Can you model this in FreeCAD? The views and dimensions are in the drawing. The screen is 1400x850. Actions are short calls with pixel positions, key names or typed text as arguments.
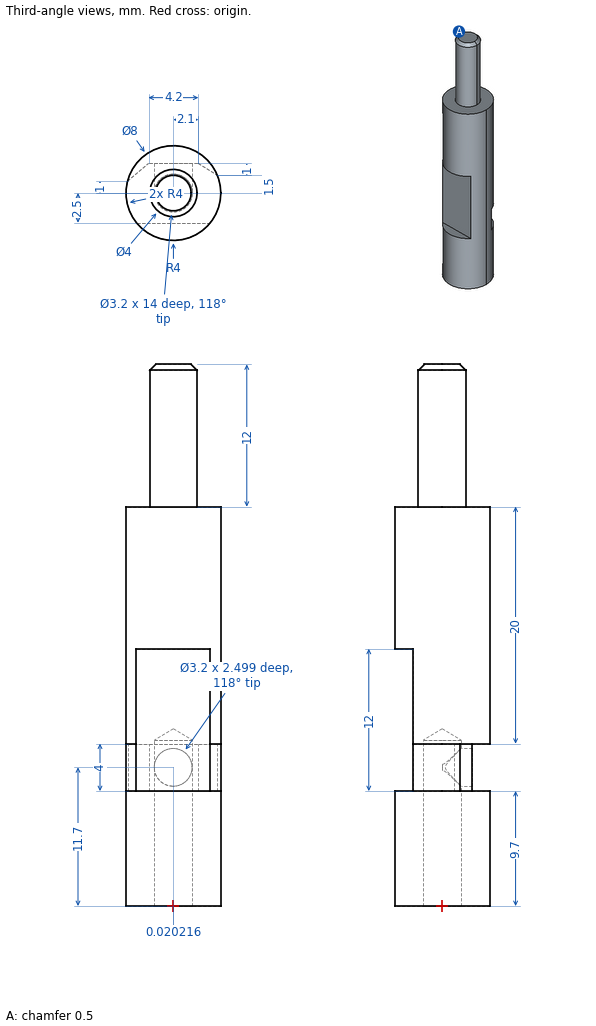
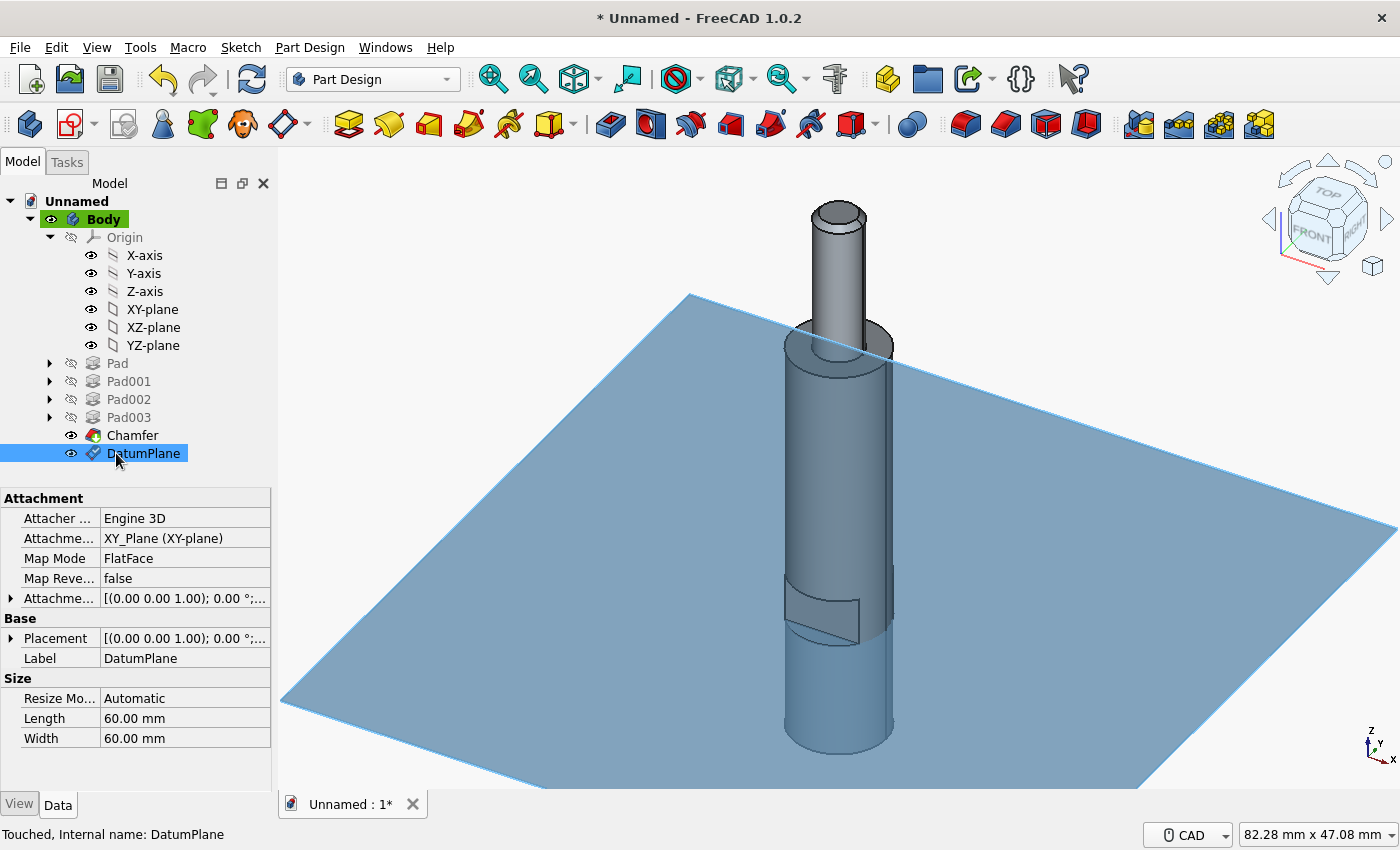
click(70, 124)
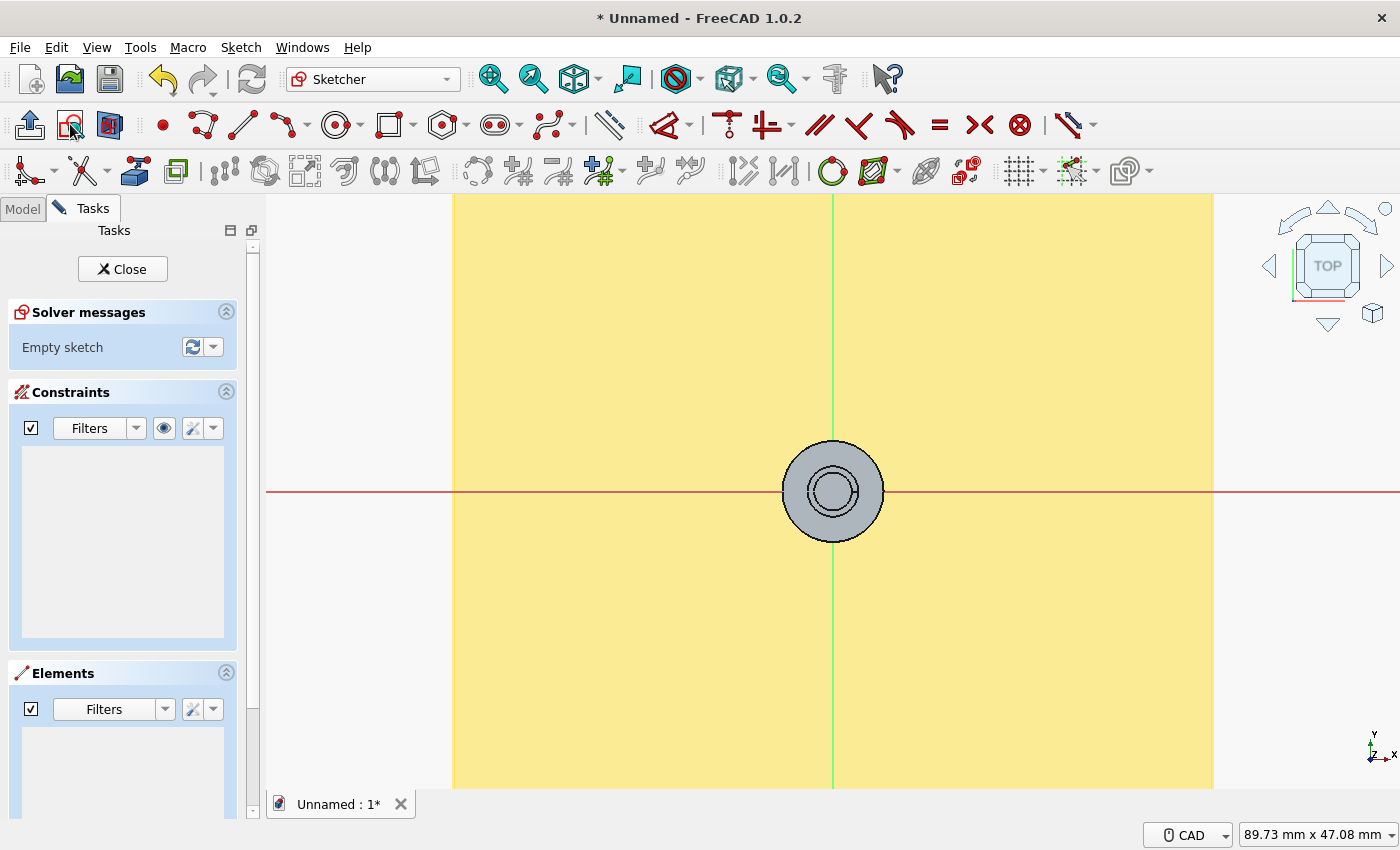
click(110, 126)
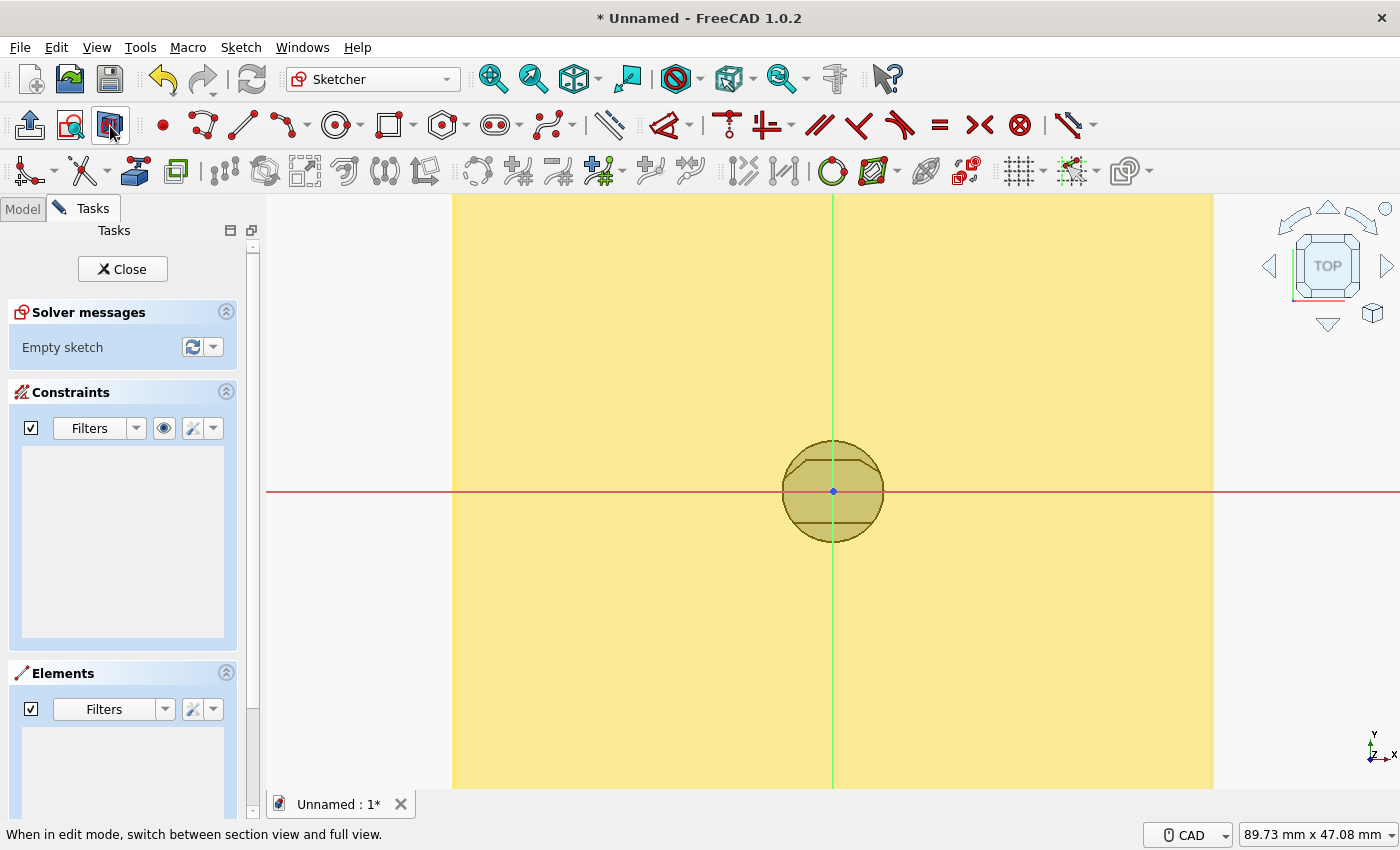
scroll(844, 521, up, 10)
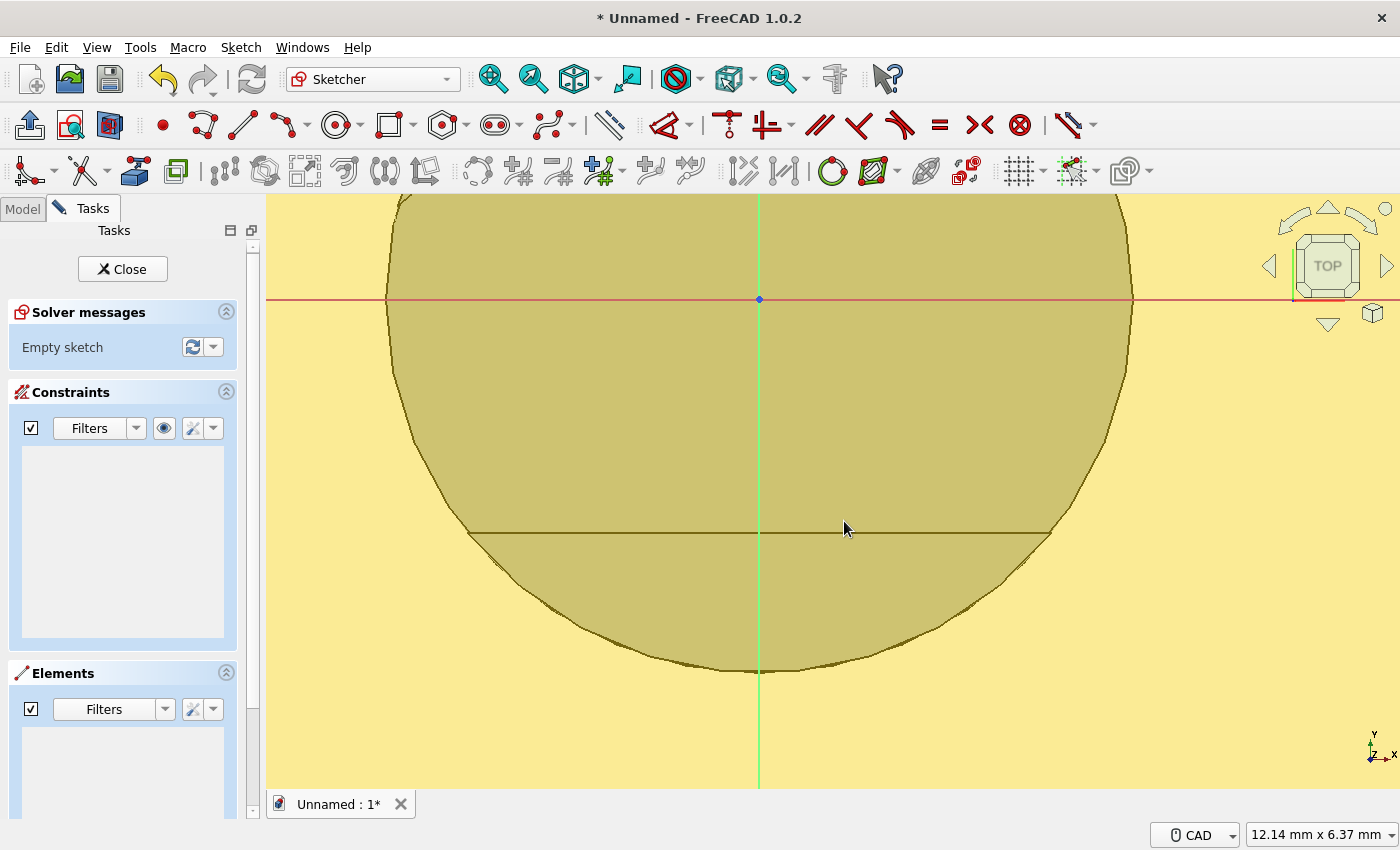
key(g)
key(l)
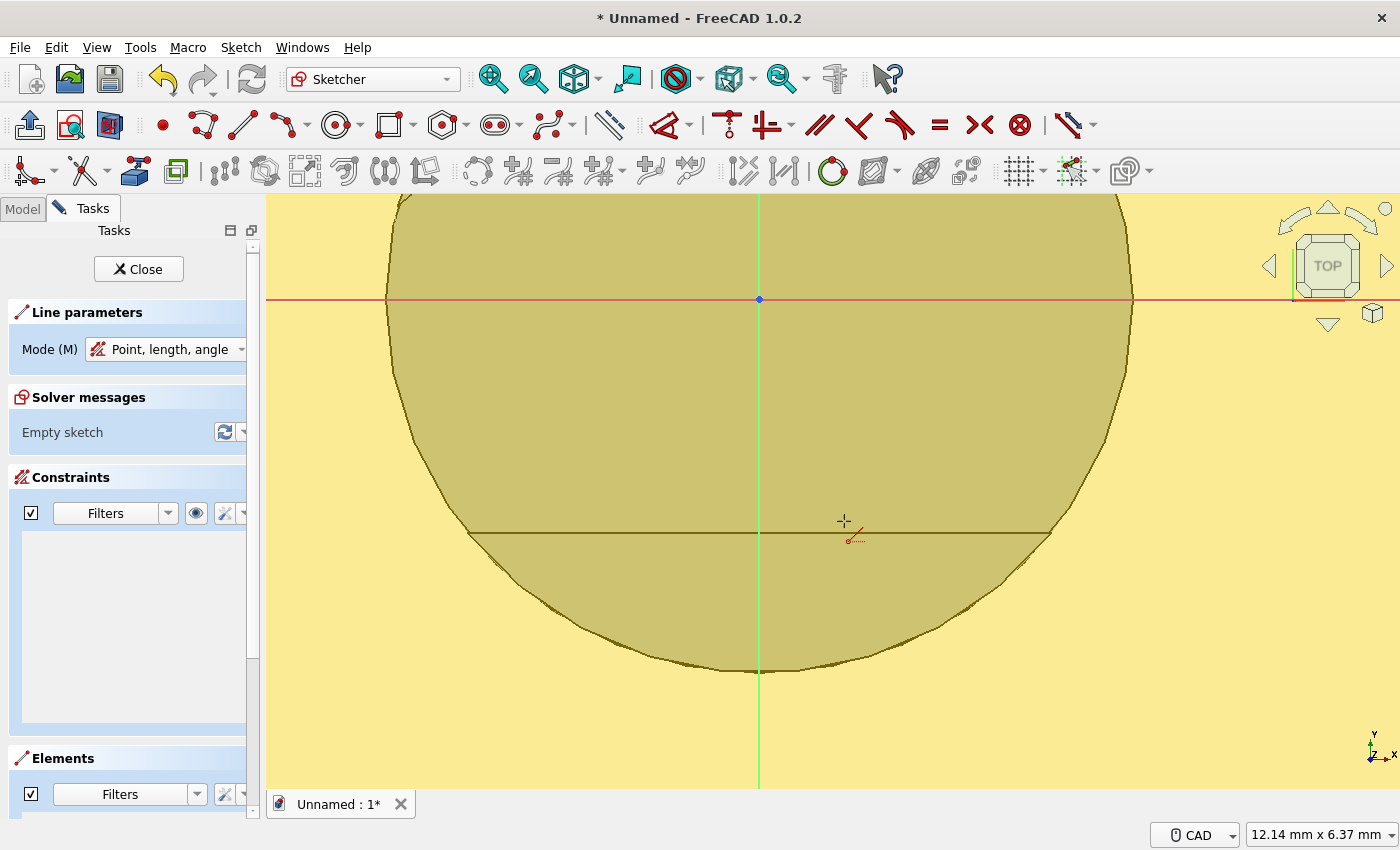
click(1051, 533)
click(468, 533)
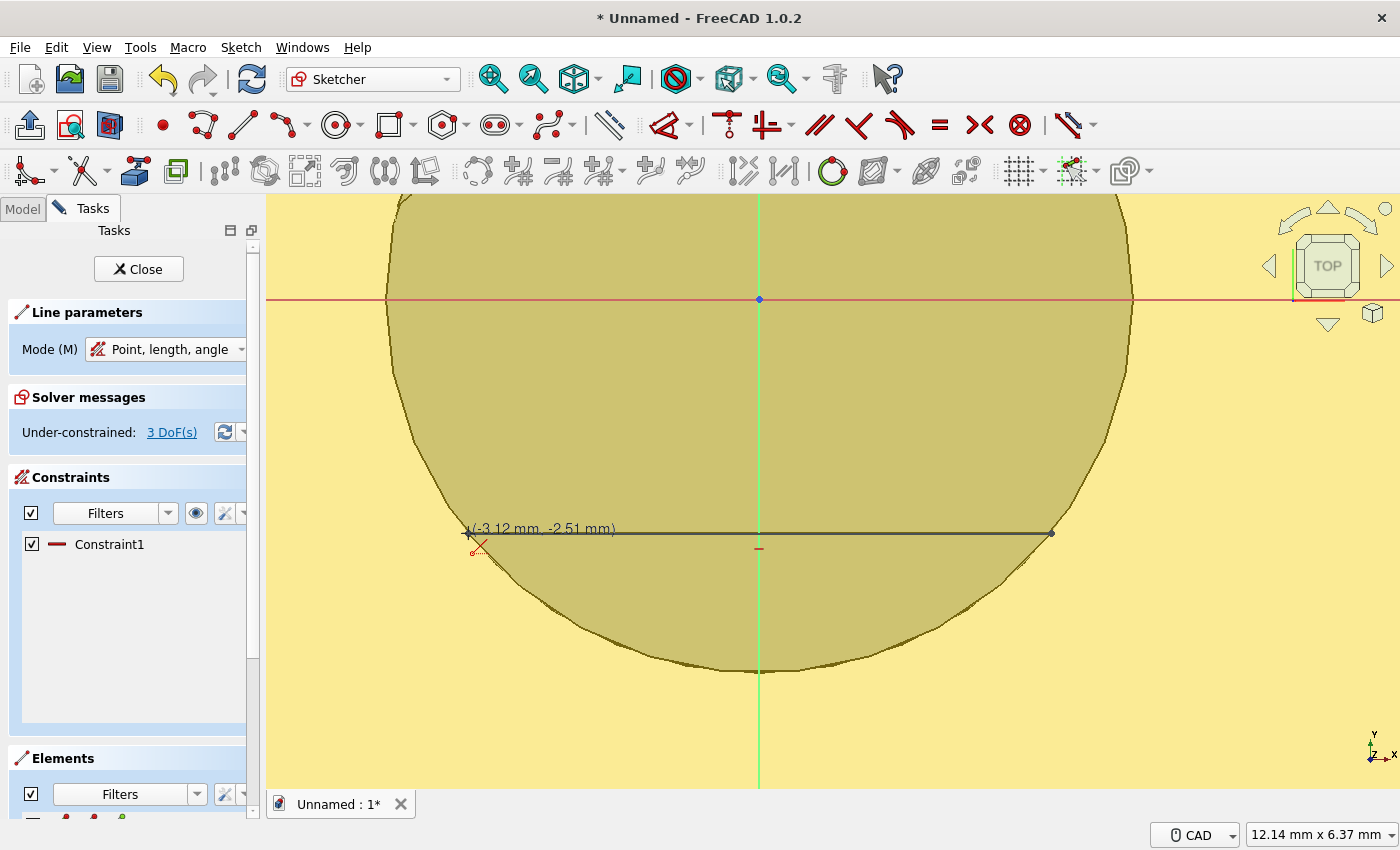
key(g)
key(3)
key(a)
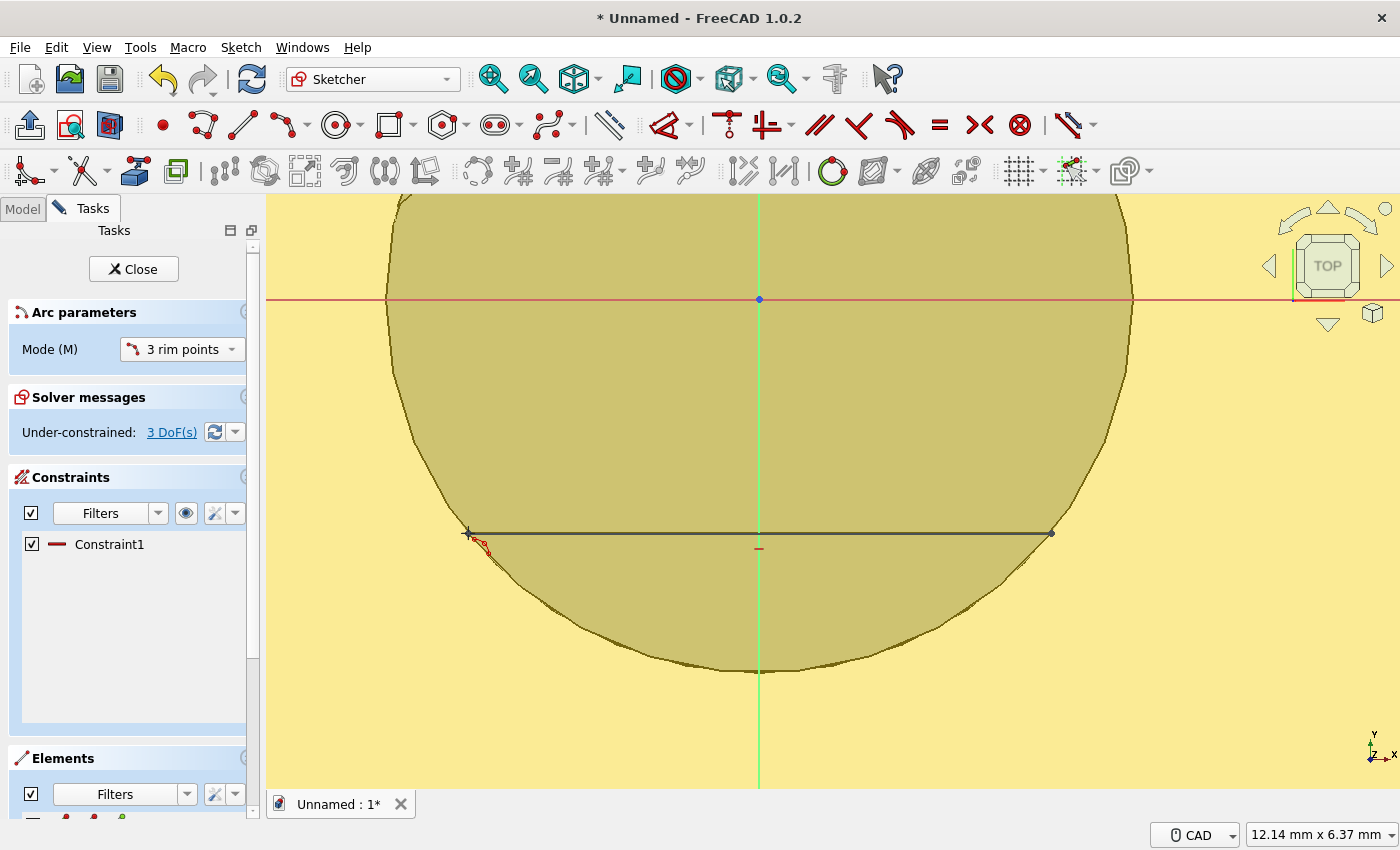
click(468, 534)
click(1051, 534)
click(693, 667)
key(Escape)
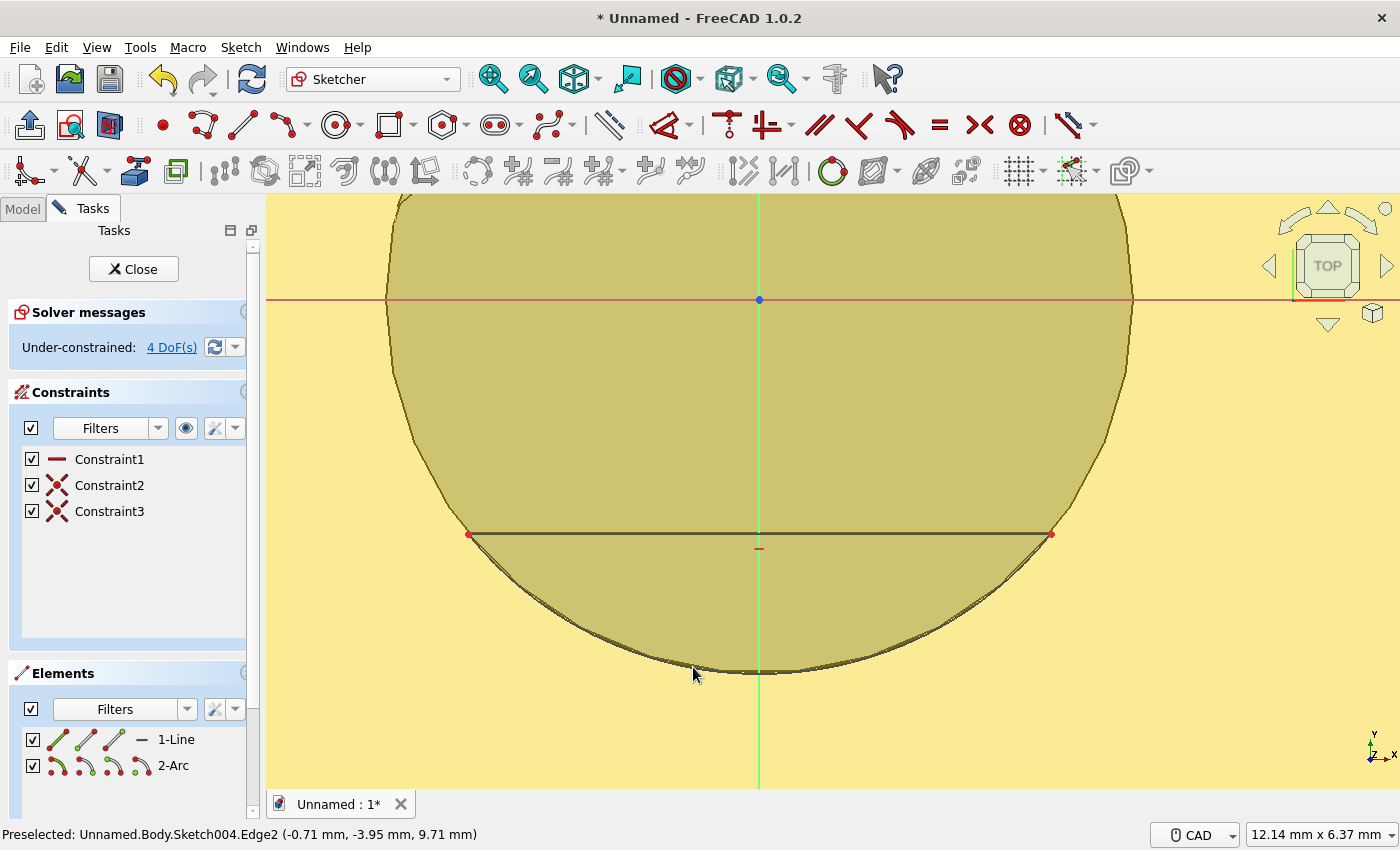
drag(749, 290, 770, 310)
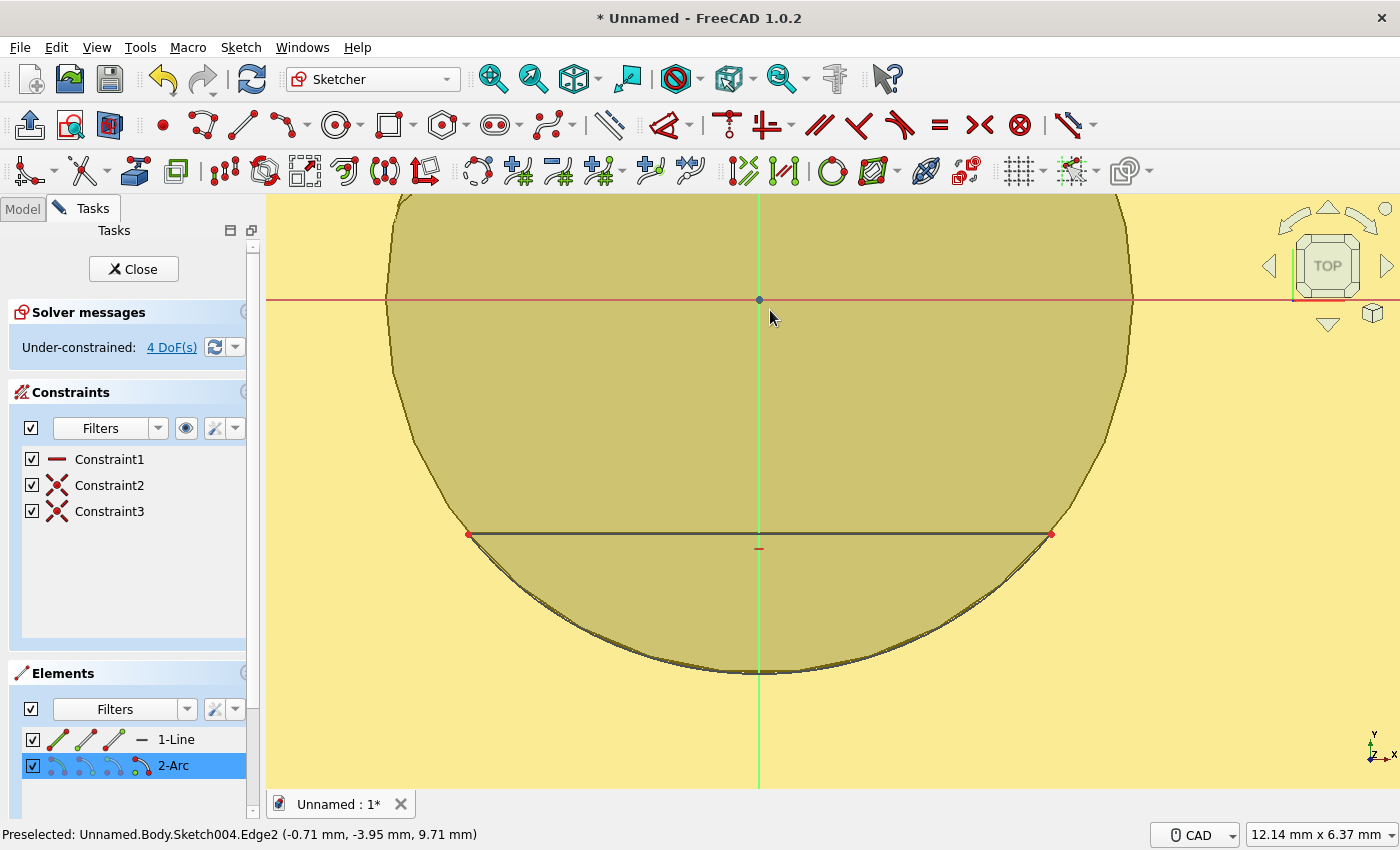
click(728, 126)